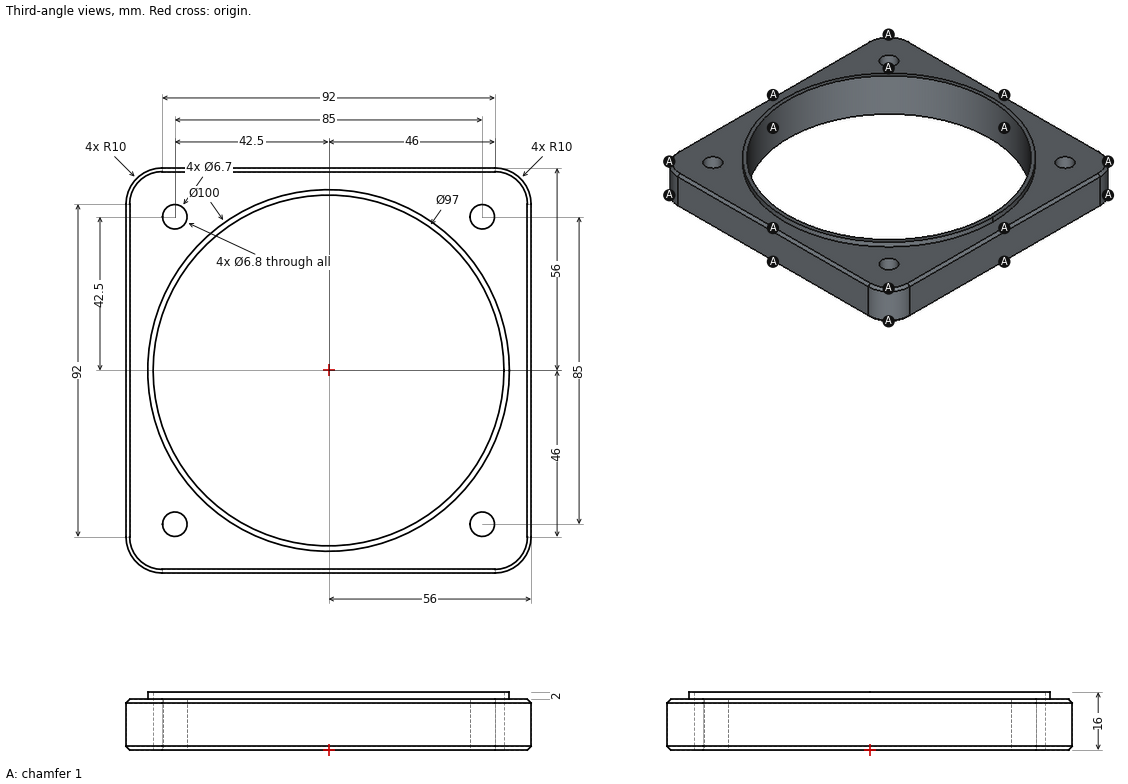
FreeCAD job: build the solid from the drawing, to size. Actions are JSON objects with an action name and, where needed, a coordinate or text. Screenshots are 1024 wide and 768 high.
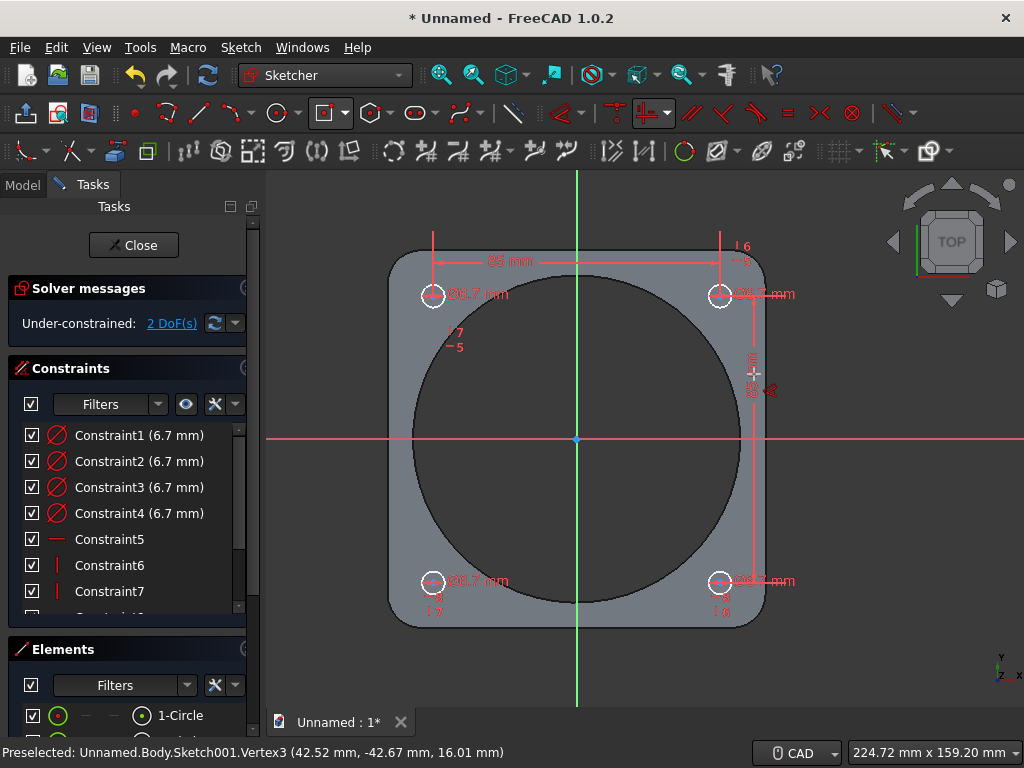
{"action": "left_click", "coordinate": [433, 296]}
{"action": "left_click", "coordinate": [505, 473]}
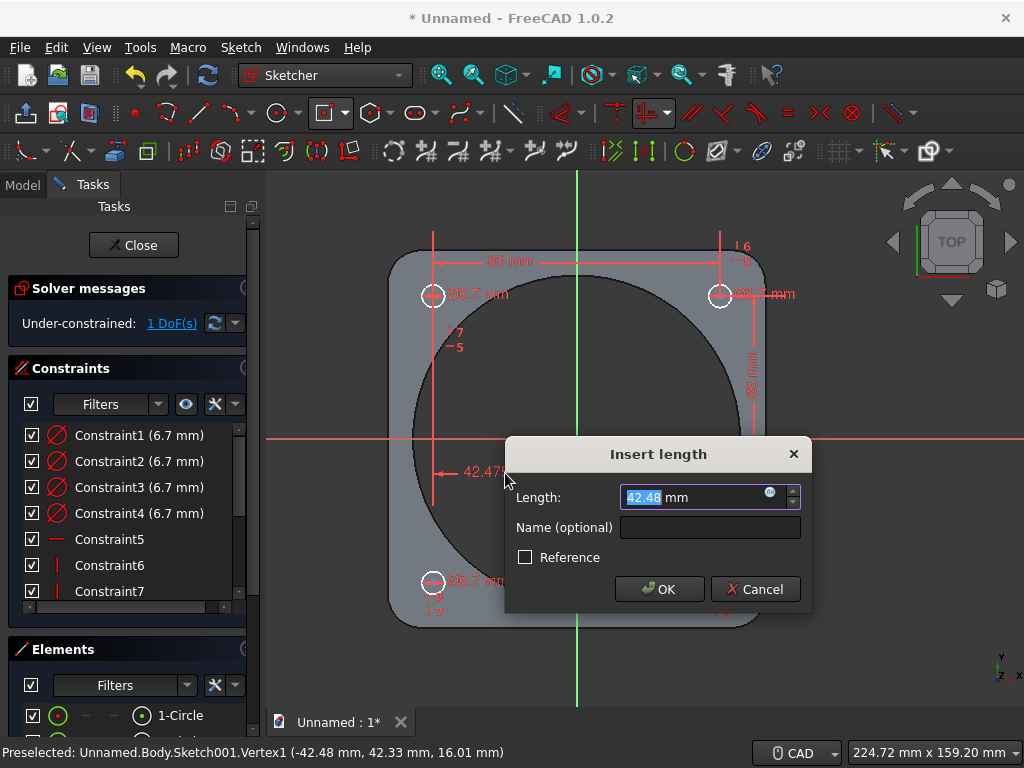
{"action": "type", "text": "42.5"}
{"action": "key", "text": "Return"}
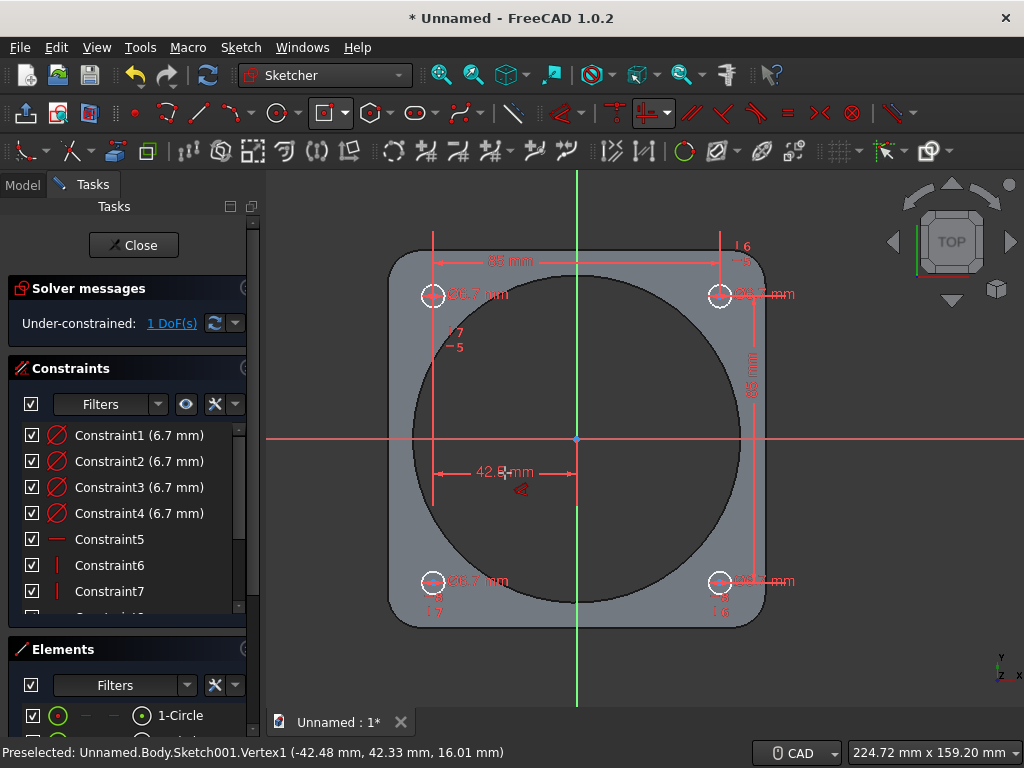
{"action": "left_click", "coordinate": [433, 296]}
{"action": "left_click", "coordinate": [399, 368]}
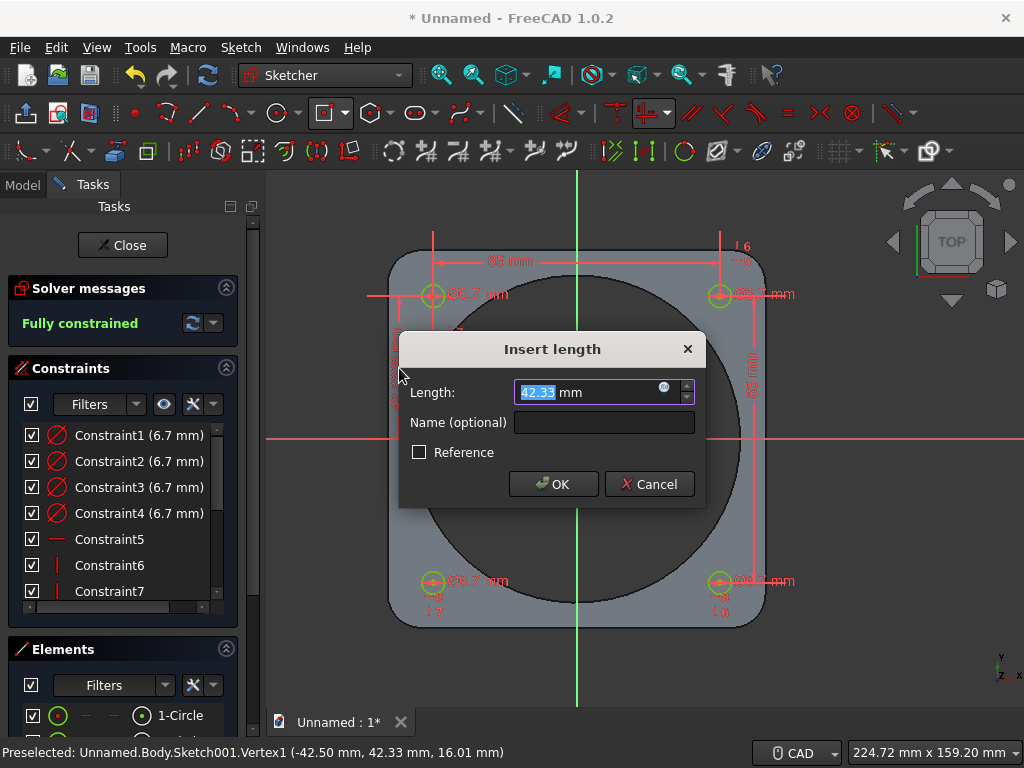
{"action": "type", "text": "42.5"}
{"action": "key", "text": "Return"}
{"action": "key", "text": "Escape"}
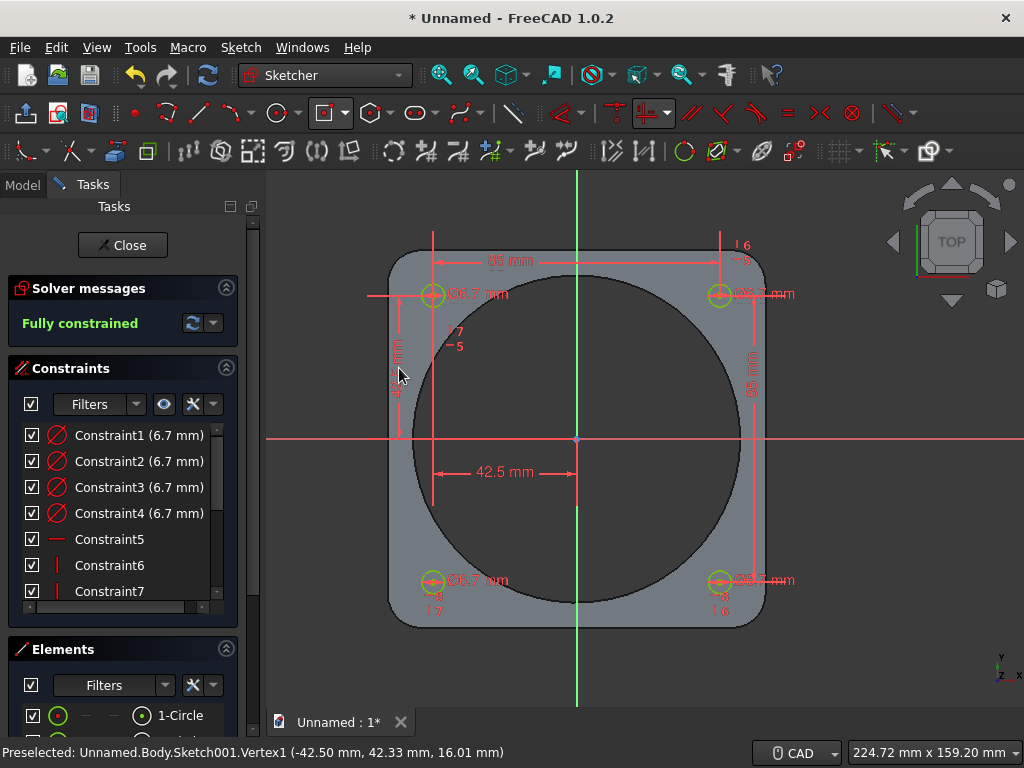
{"action": "left_click", "coordinate": [123, 245]}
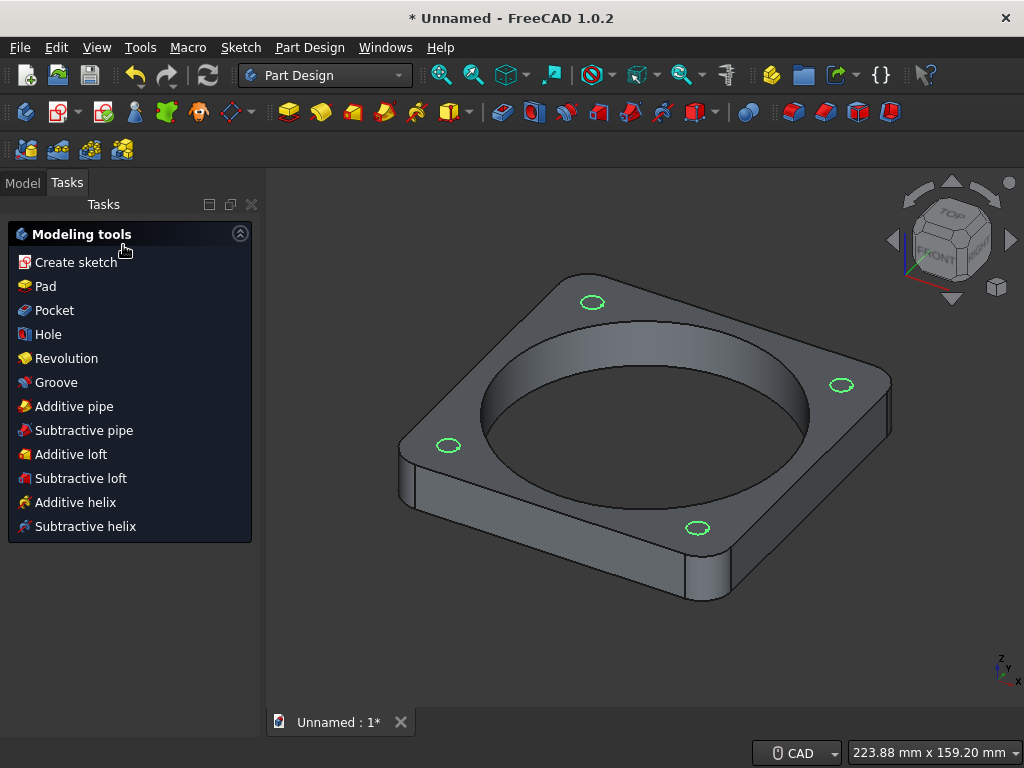
{"action": "left_click", "coordinate": [504, 112]}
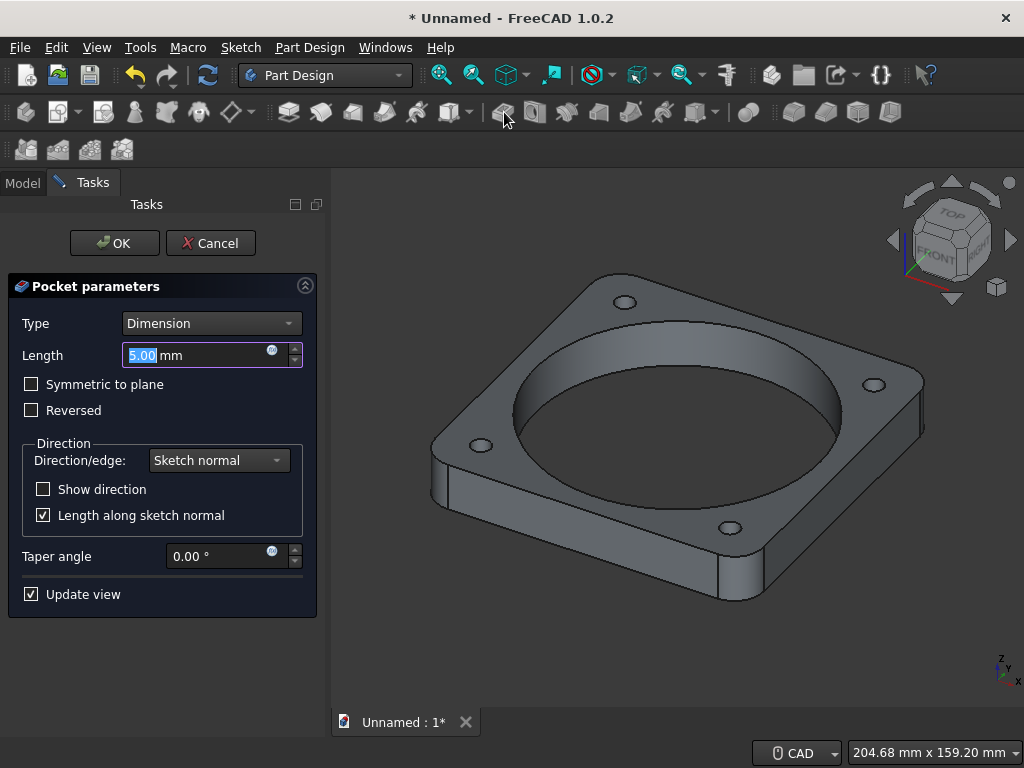
{"action": "left_click", "coordinate": [212, 324]}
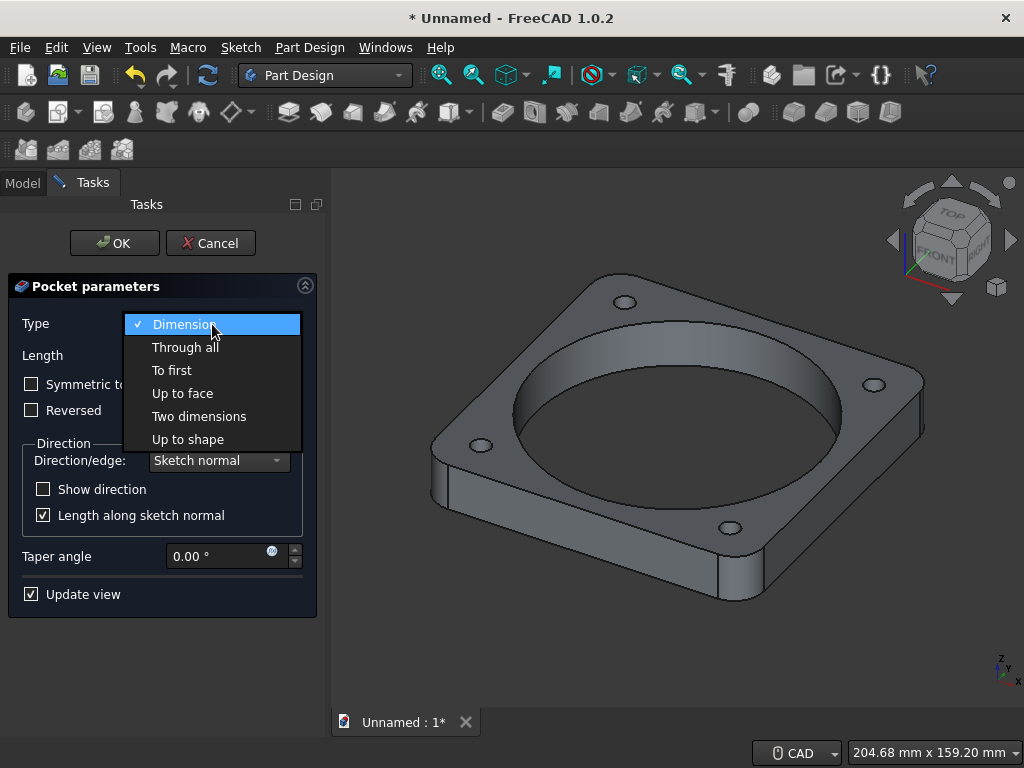
{"action": "left_click", "coordinate": [212, 348]}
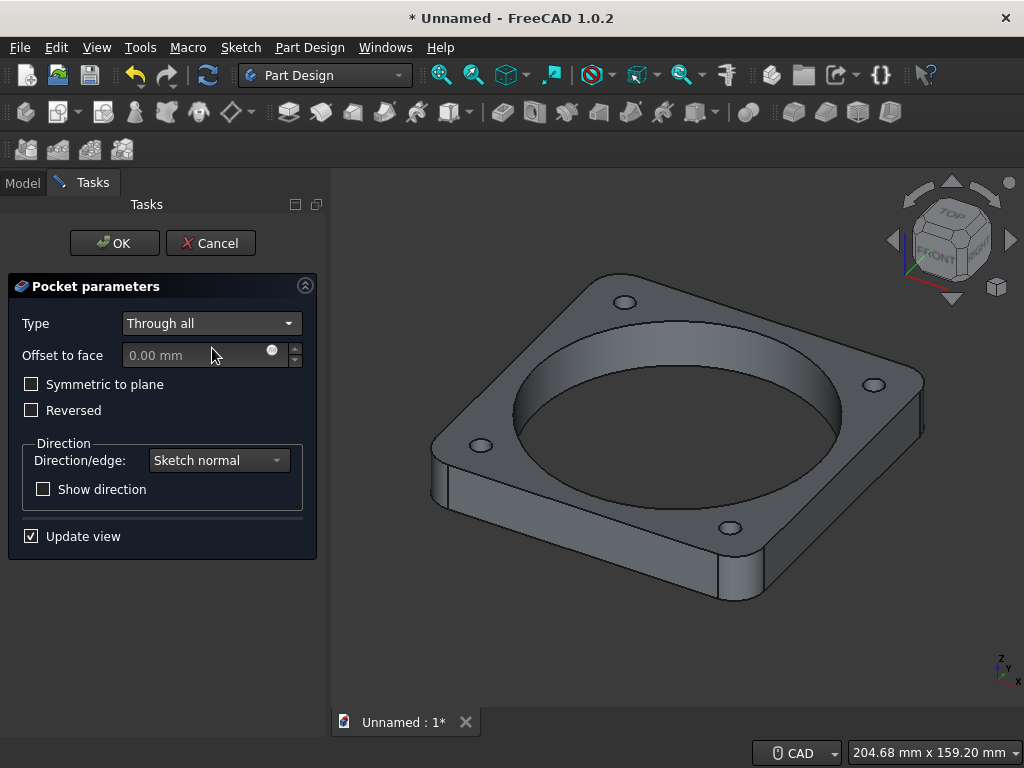
{"action": "left_click", "coordinate": [115, 243]}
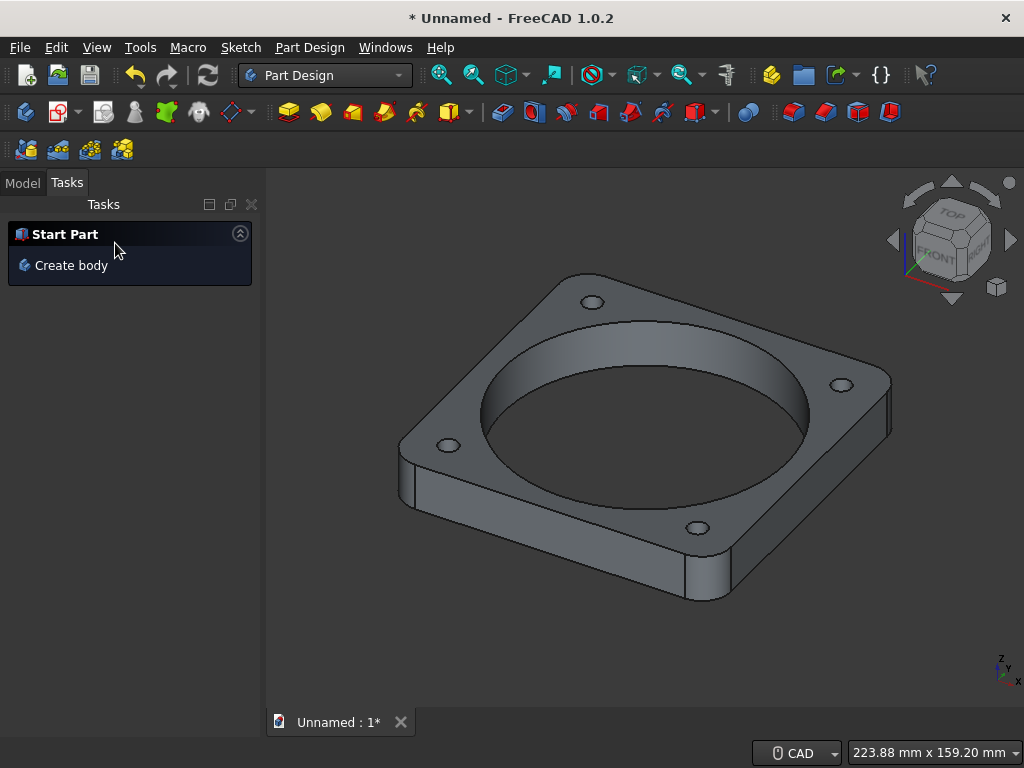
{"action": "left_click", "coordinate": [558, 314]}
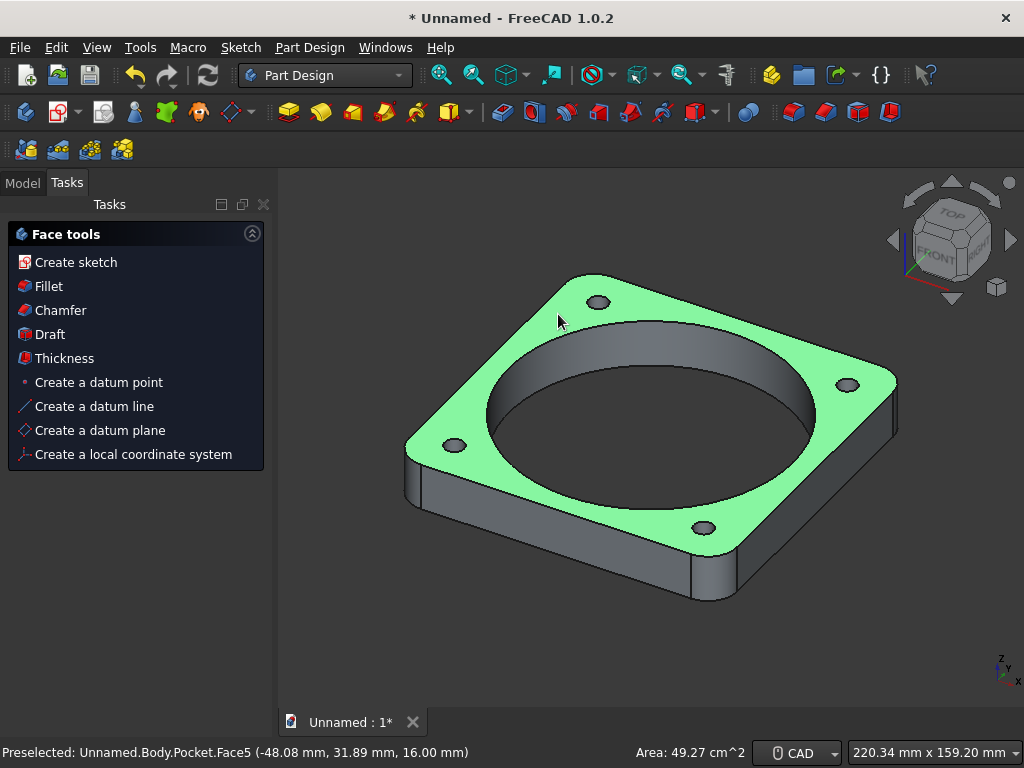
{"action": "left_click", "coordinate": [58, 112]}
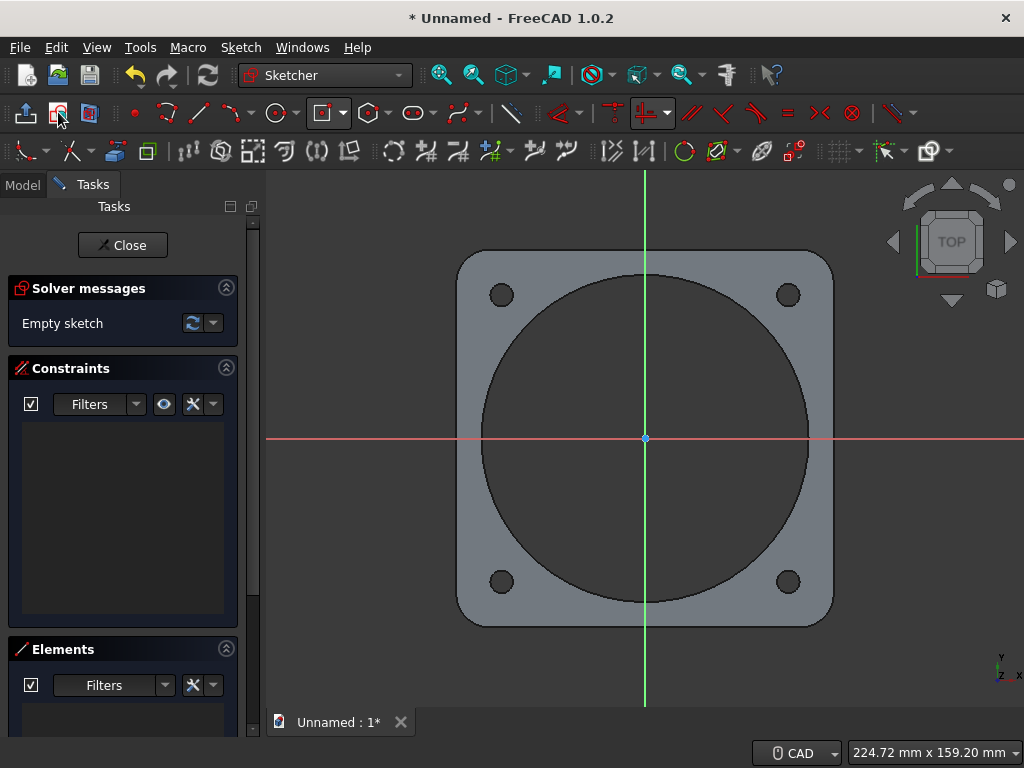
{"action": "left_click", "coordinate": [276, 114]}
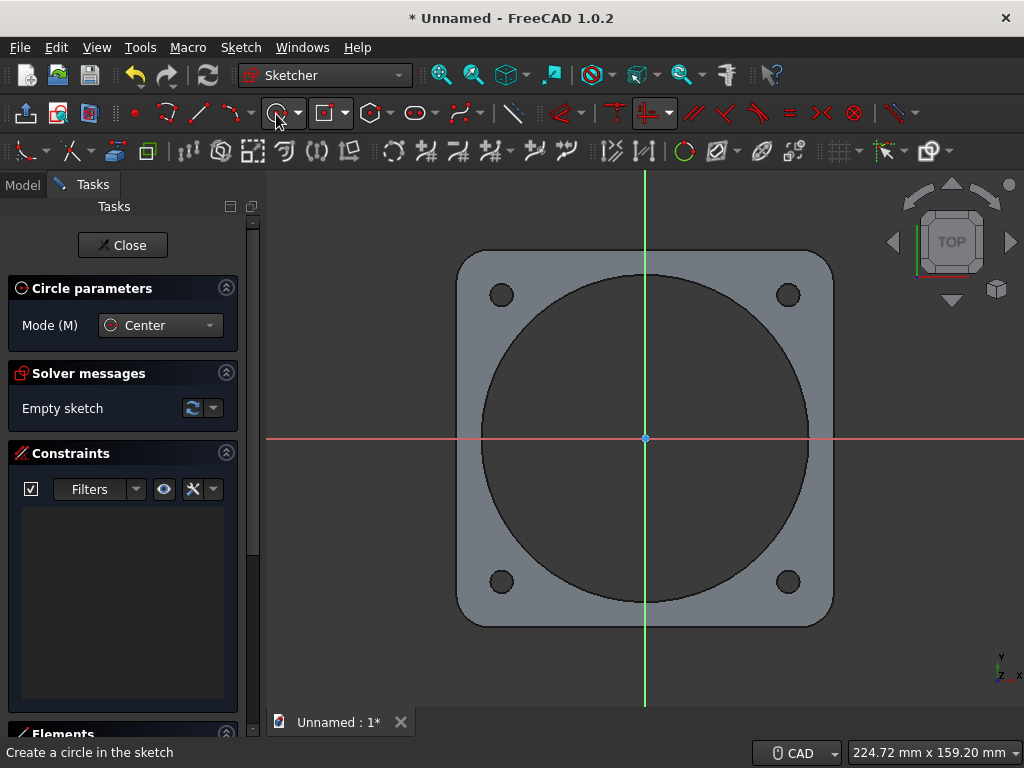
{"action": "scroll", "coordinate": [502, 295], "scroll_direction": "up", "scroll_amount": 4}